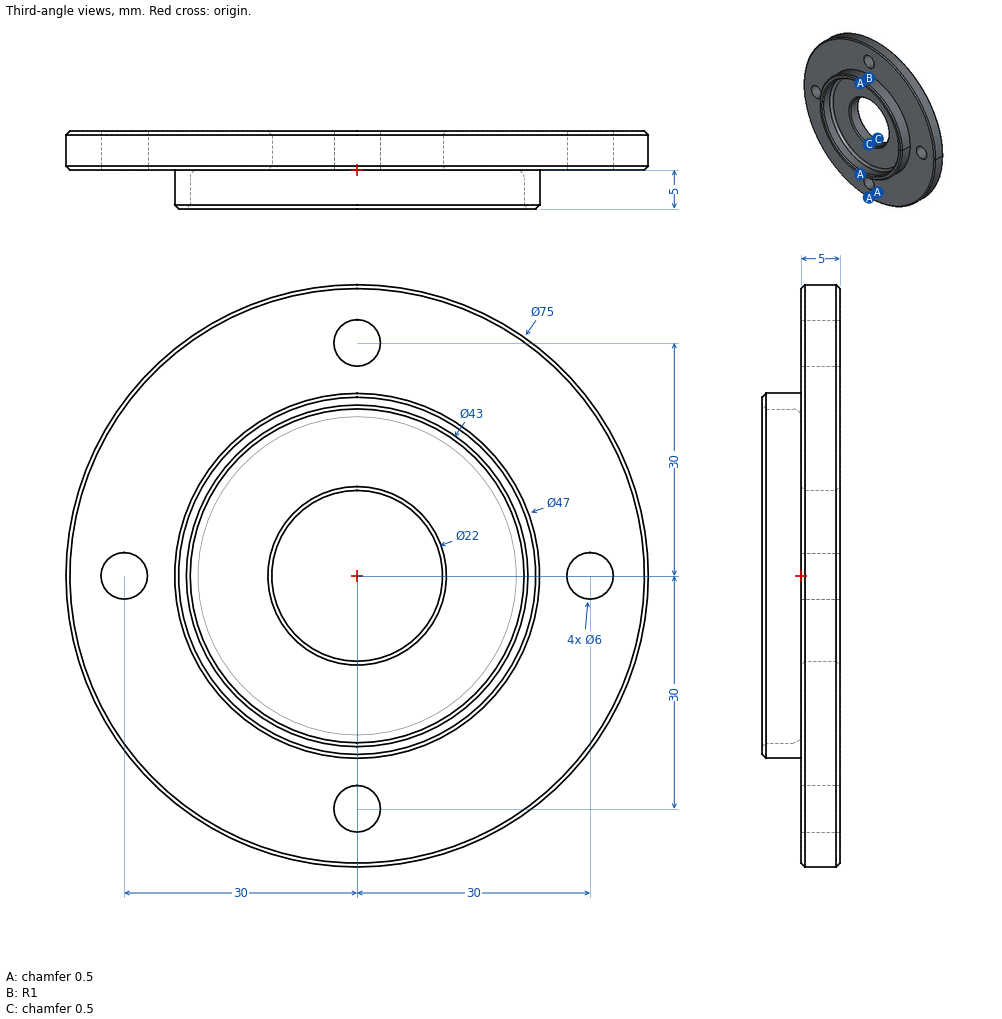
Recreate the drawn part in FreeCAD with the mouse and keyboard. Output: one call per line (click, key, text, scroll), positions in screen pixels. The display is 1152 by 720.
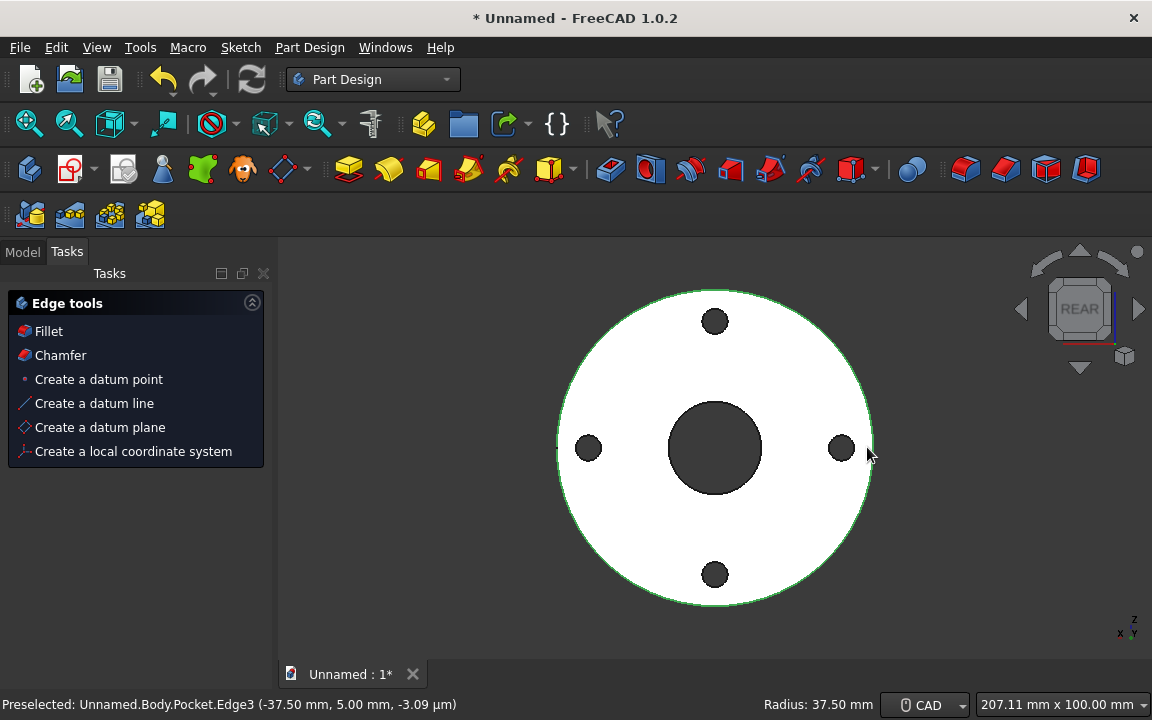
key(0)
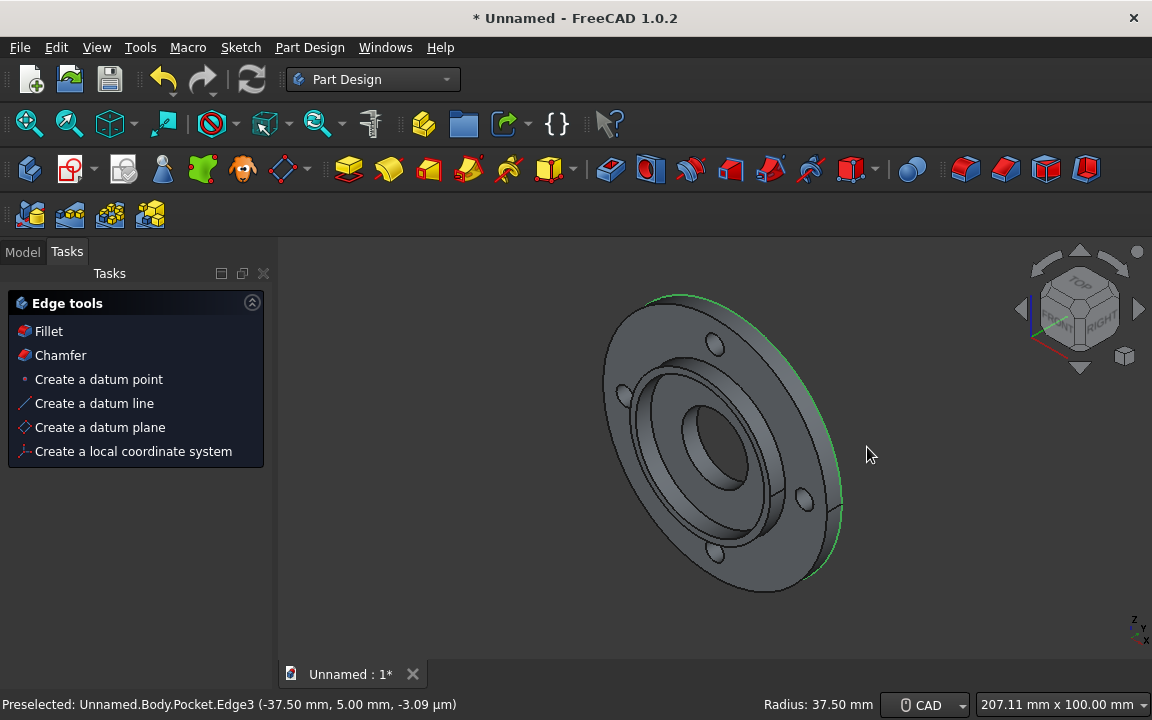
click(678, 366, ctrl)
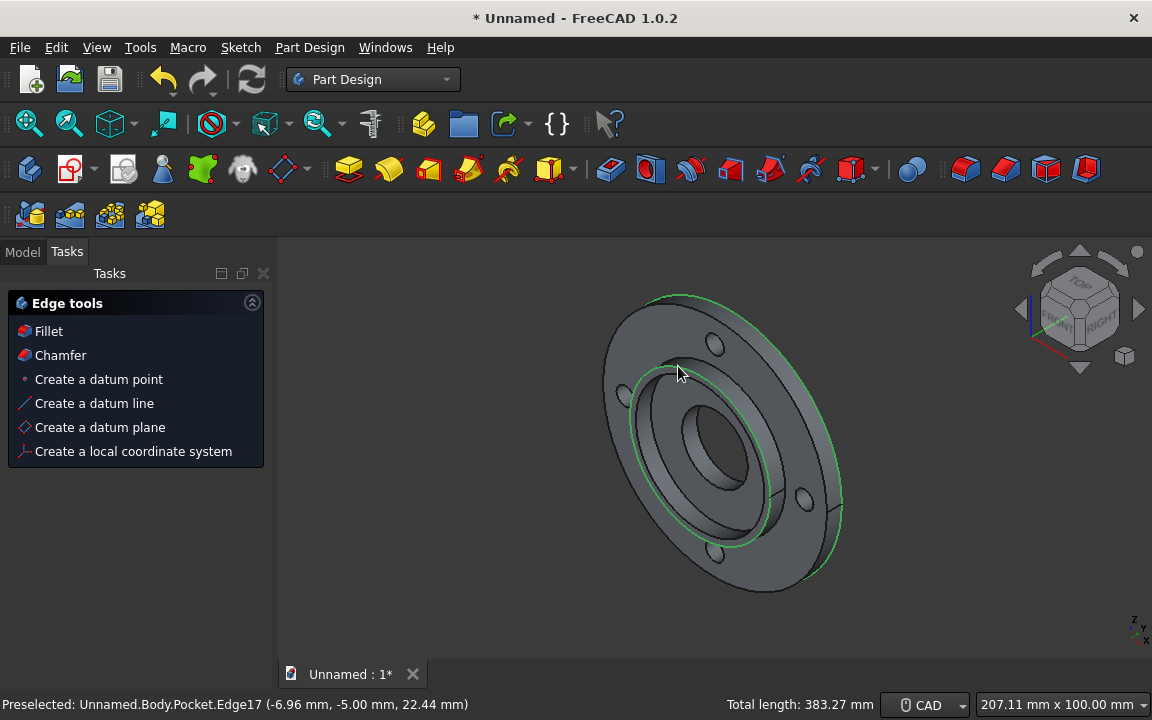
click(636, 419, ctrl)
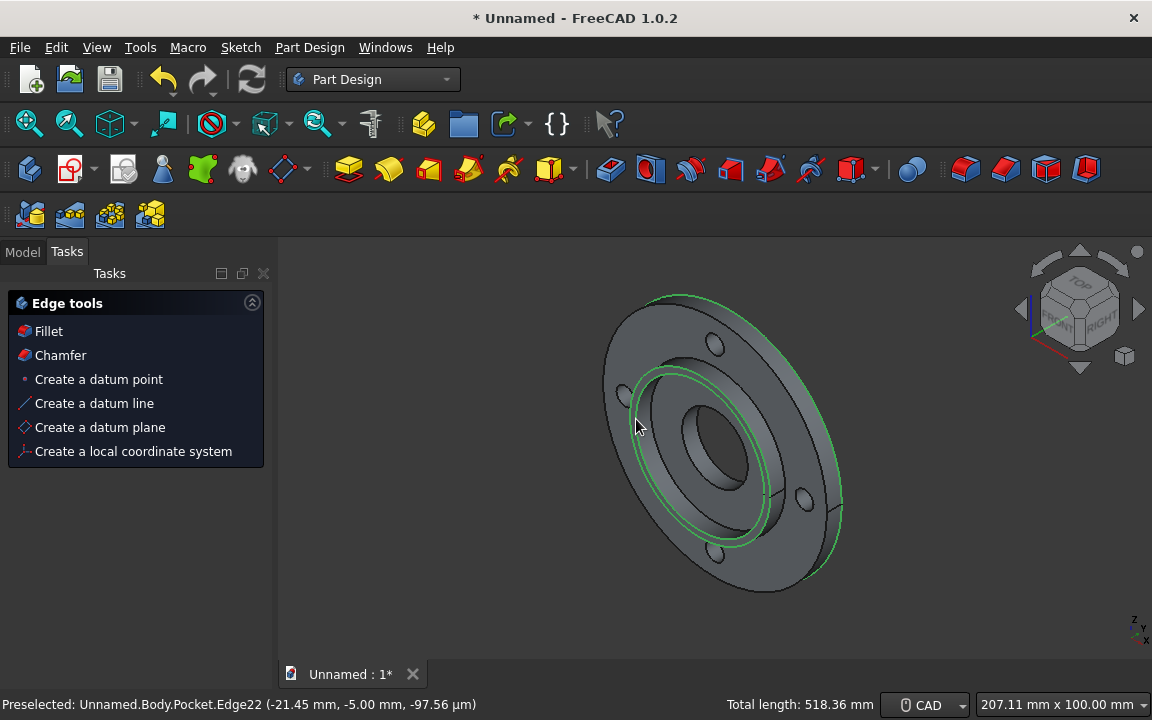
click(624, 319, ctrl)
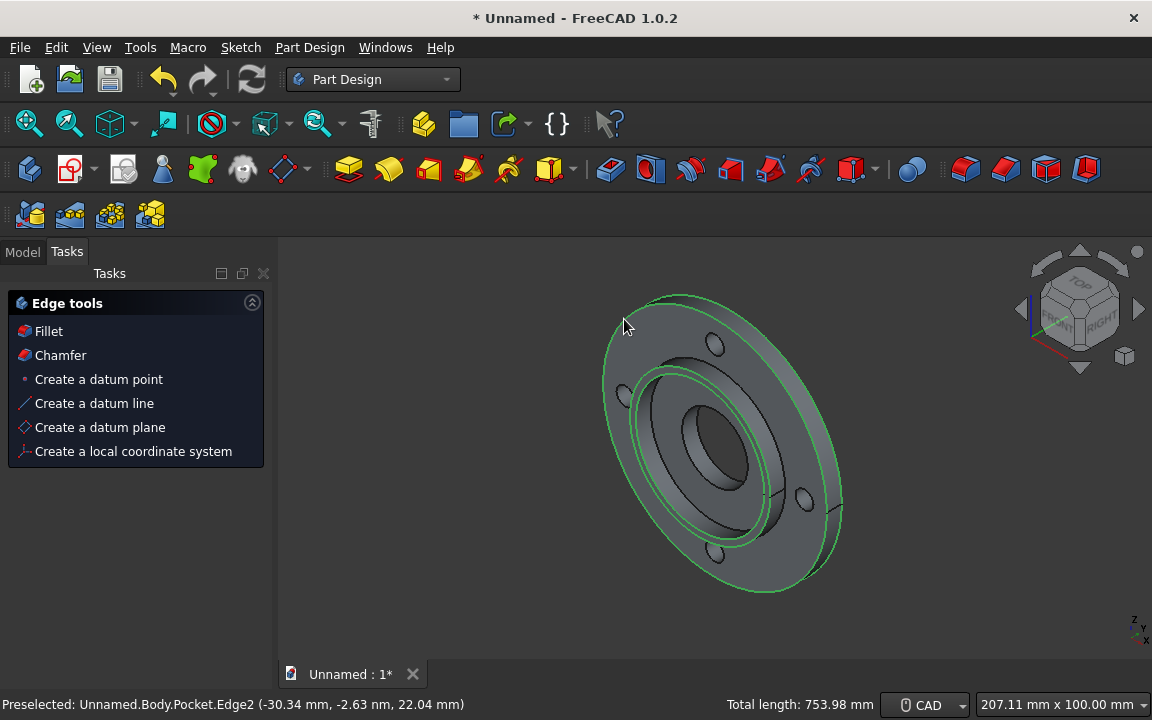
click(1006, 170)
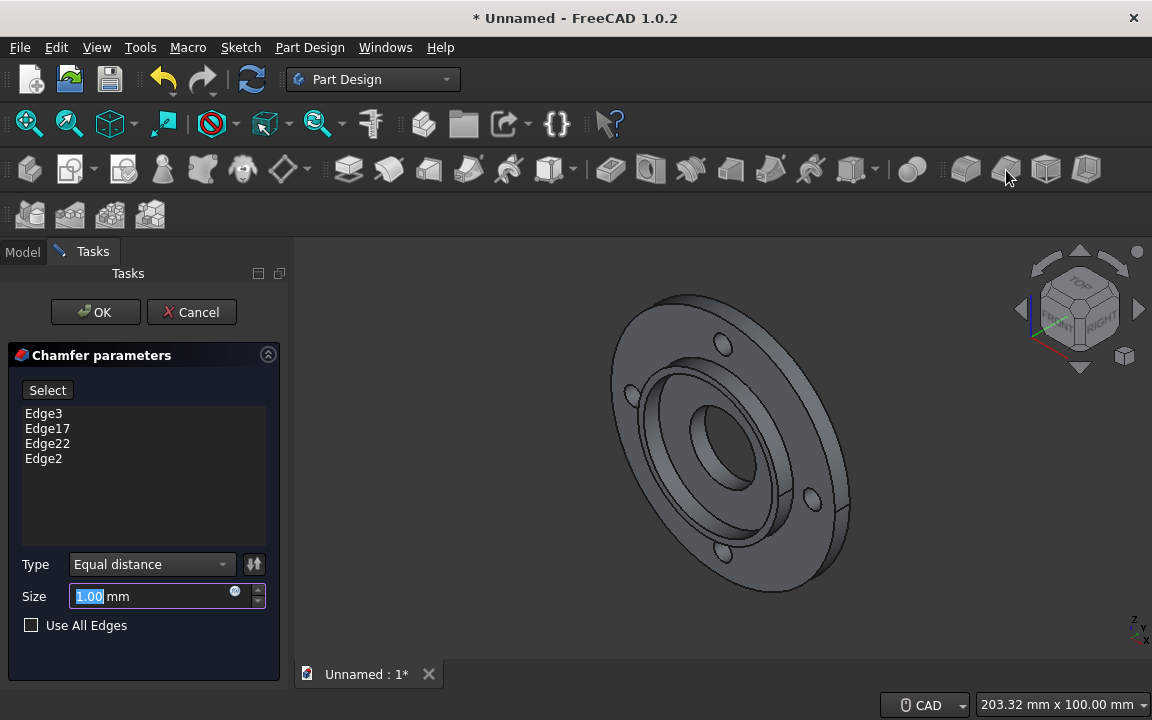
text(0.5)
key(Tab)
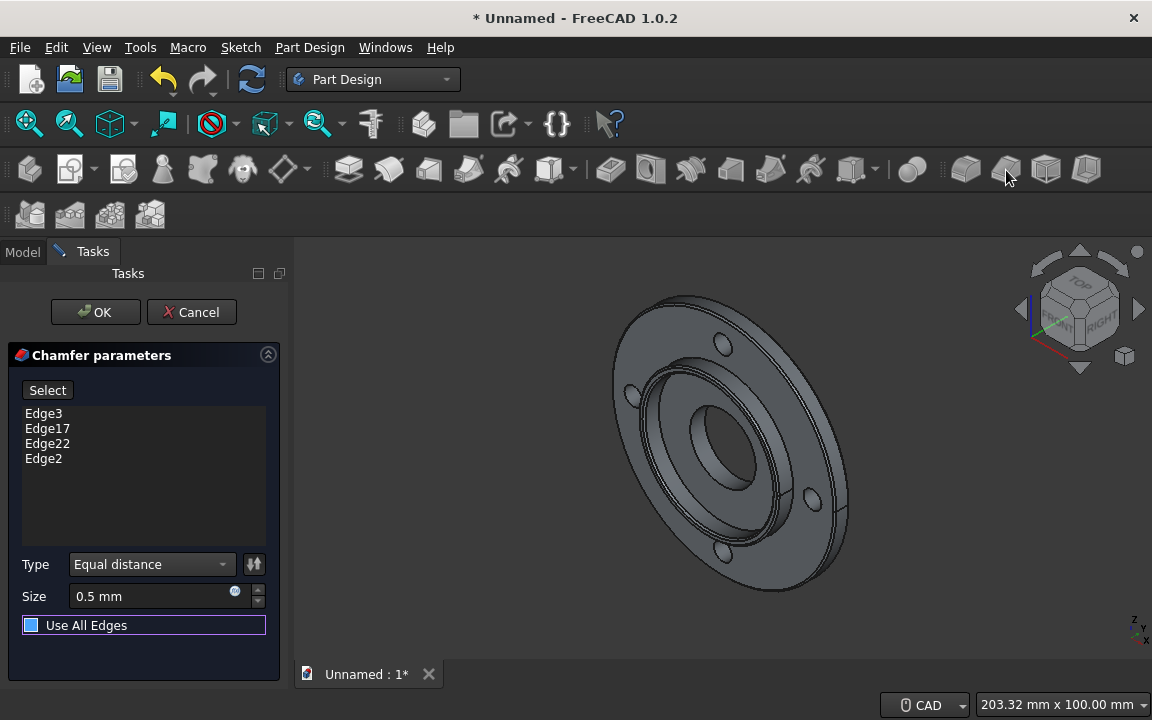
click(96, 312)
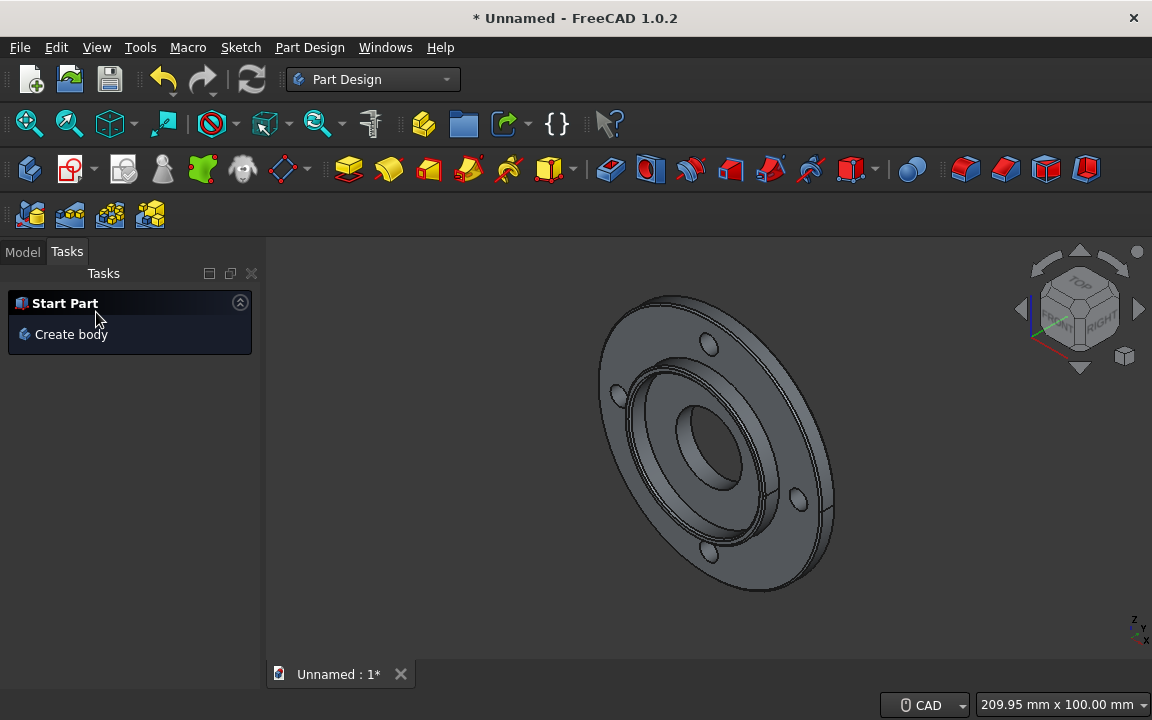
key(2)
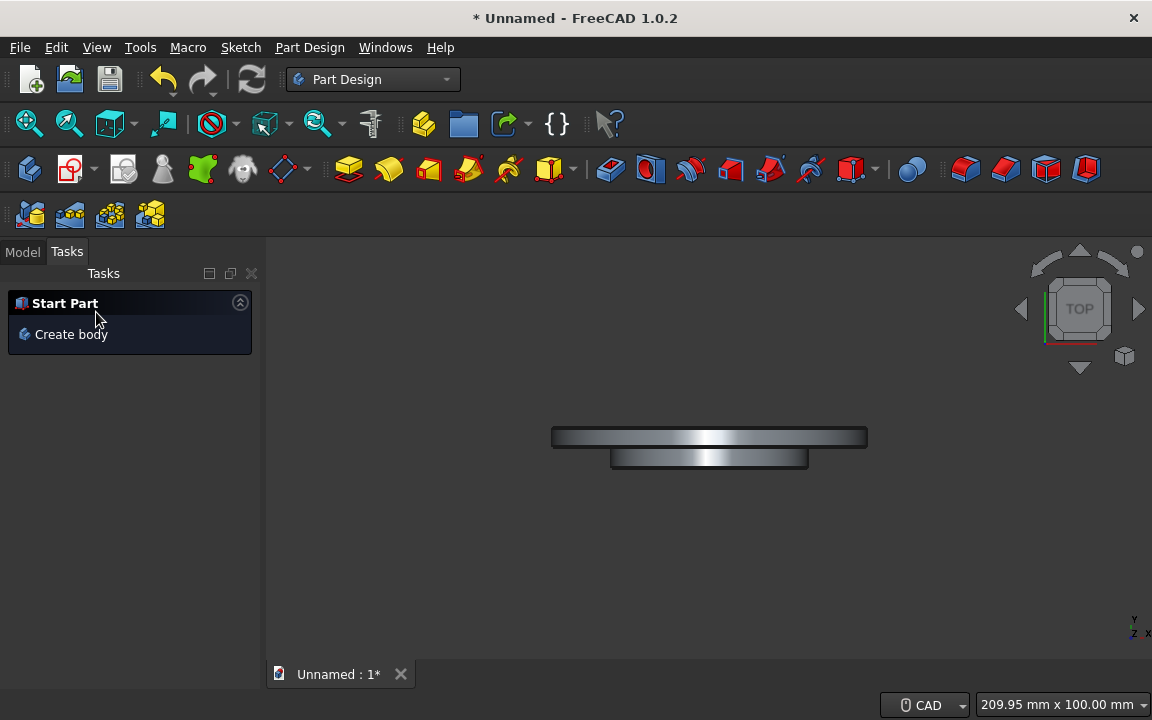
click(30, 124)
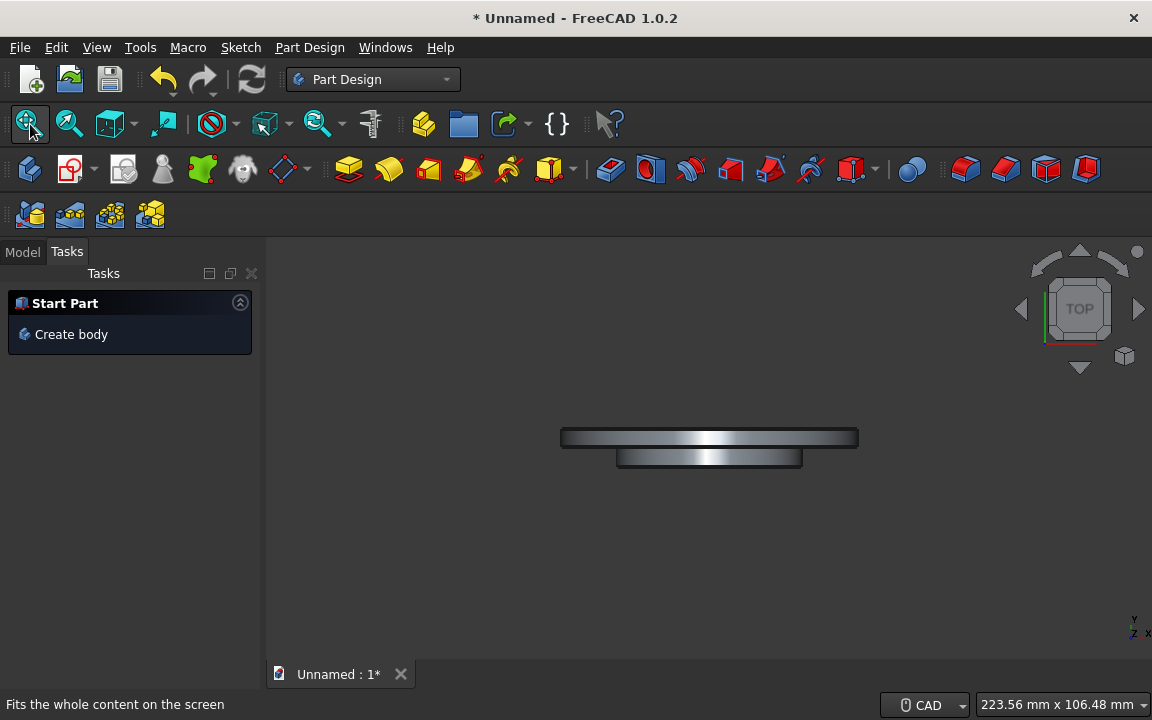
key(0)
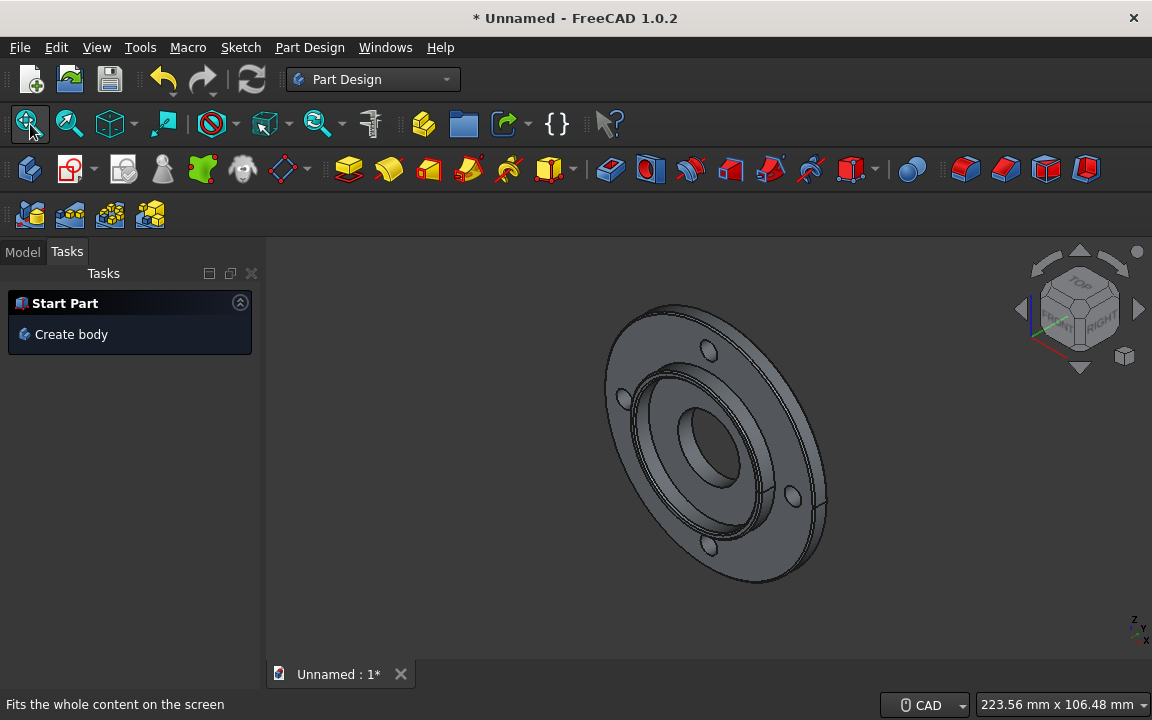
key(1)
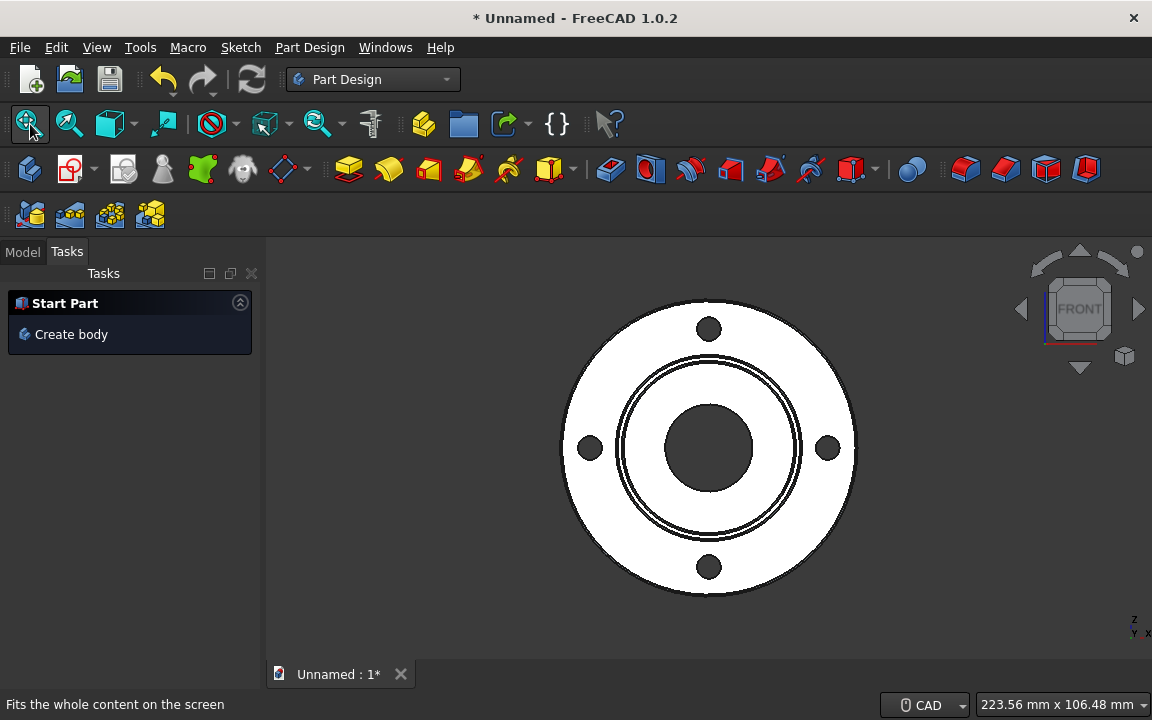
key(3)